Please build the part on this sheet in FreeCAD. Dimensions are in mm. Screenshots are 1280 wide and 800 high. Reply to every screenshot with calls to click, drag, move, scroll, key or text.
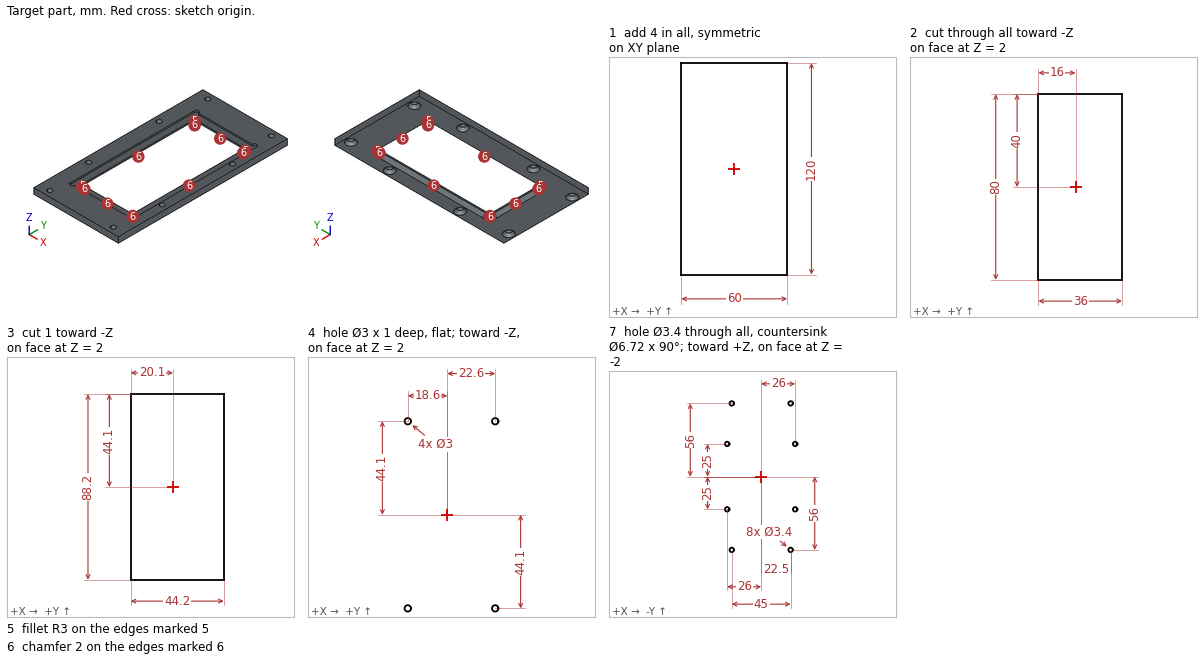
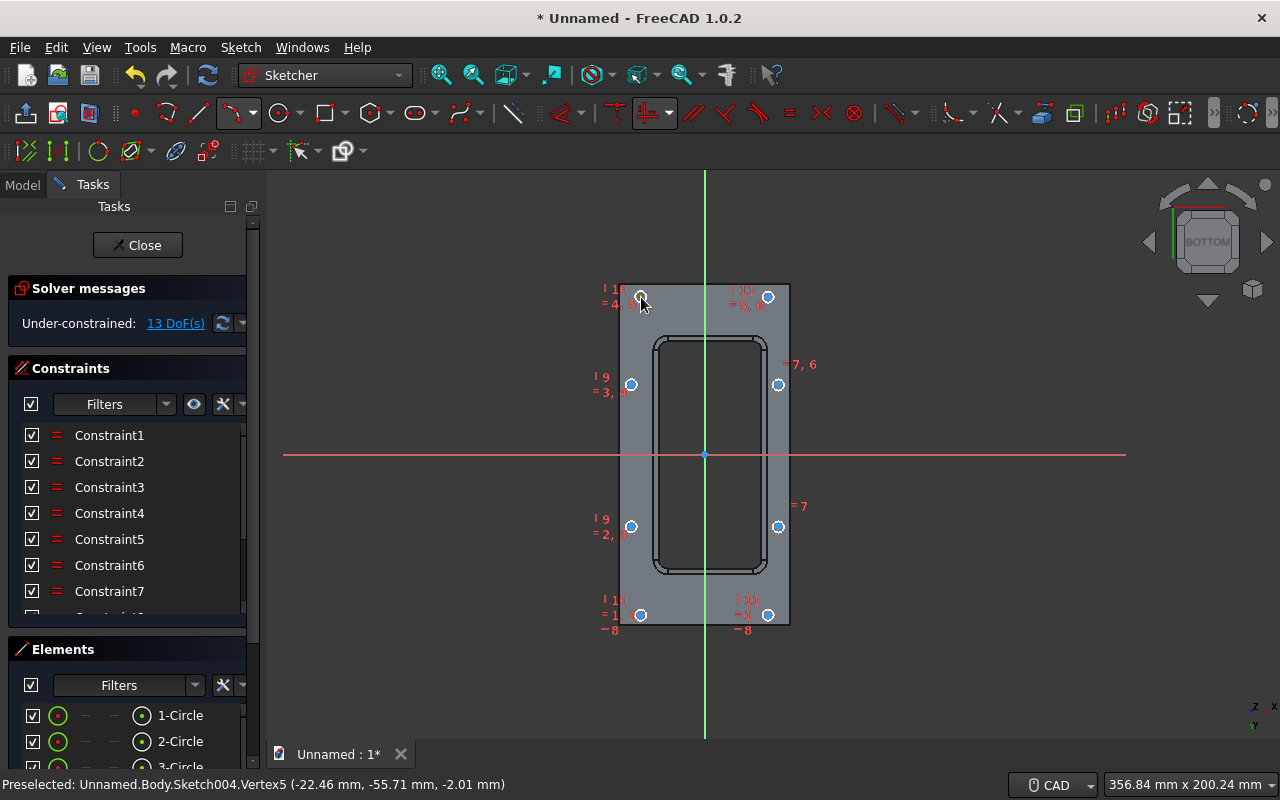
click(768, 297)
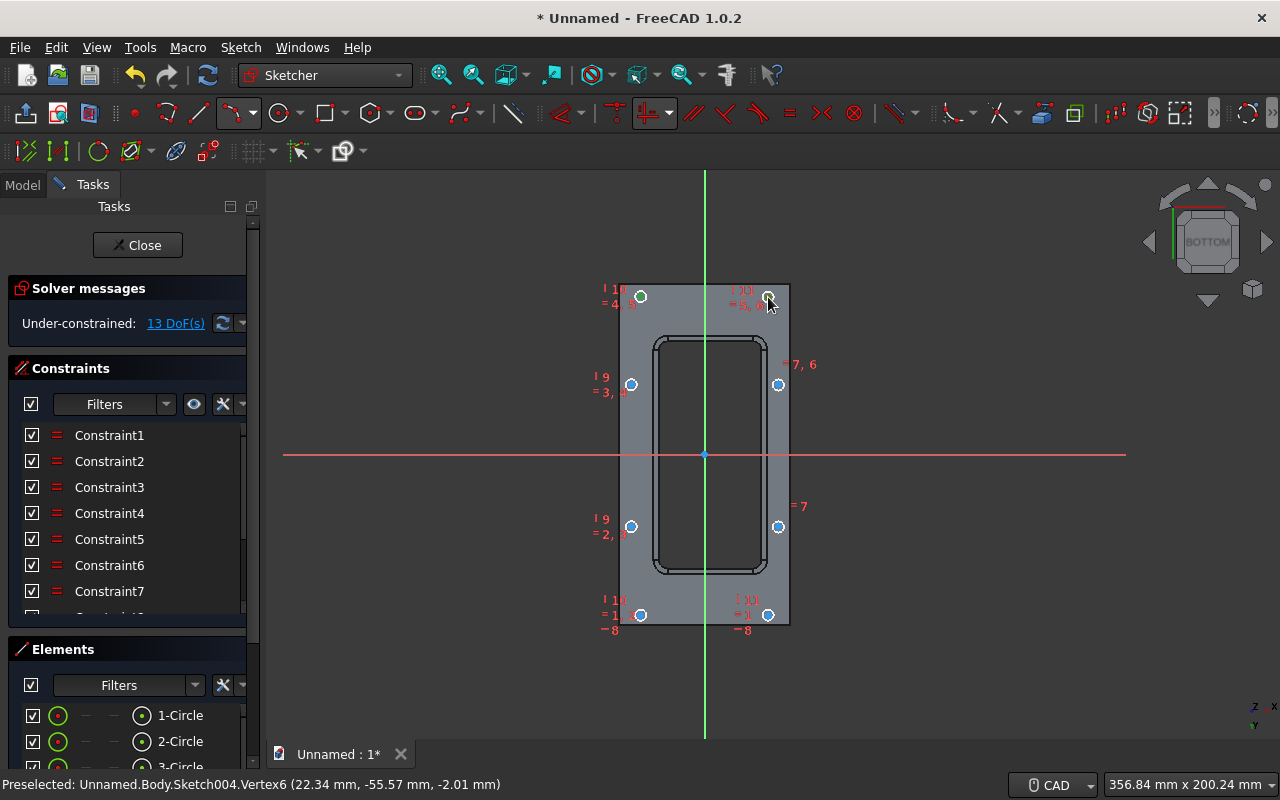
key(h)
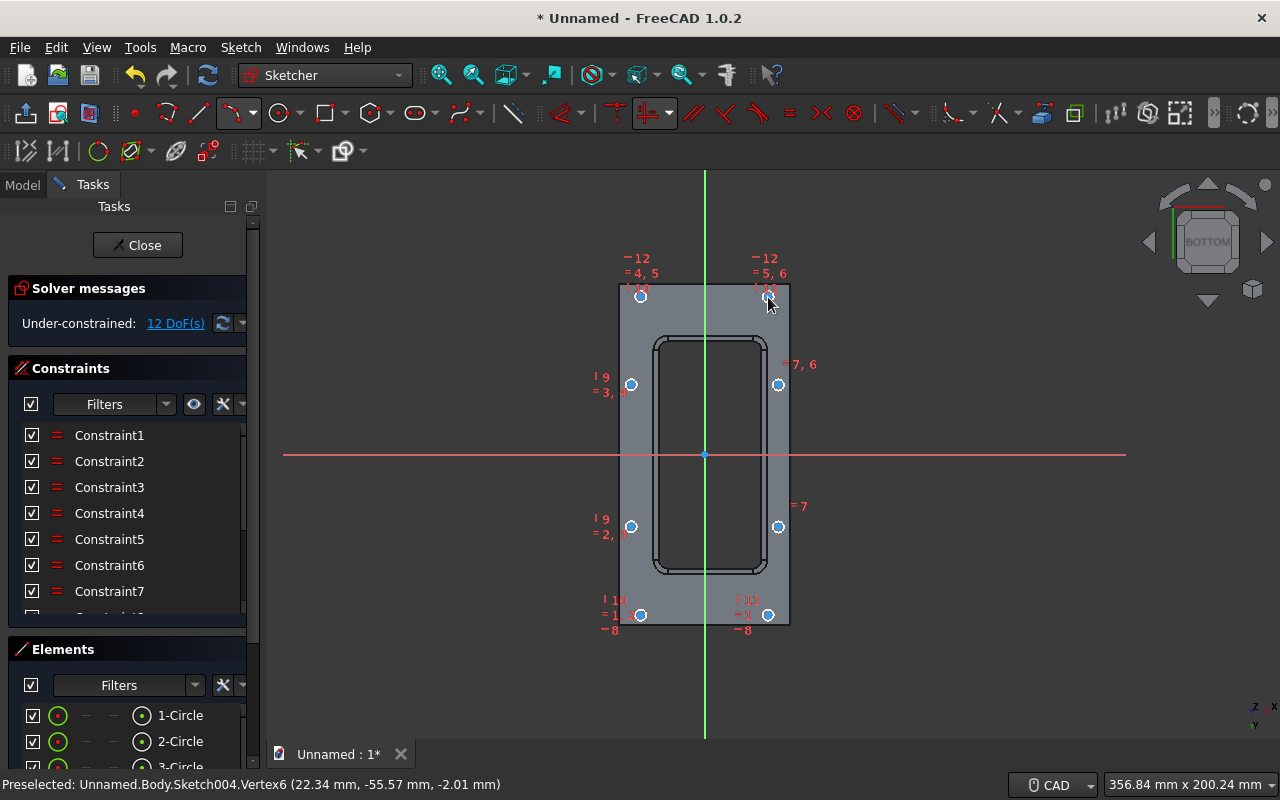
click(631, 385)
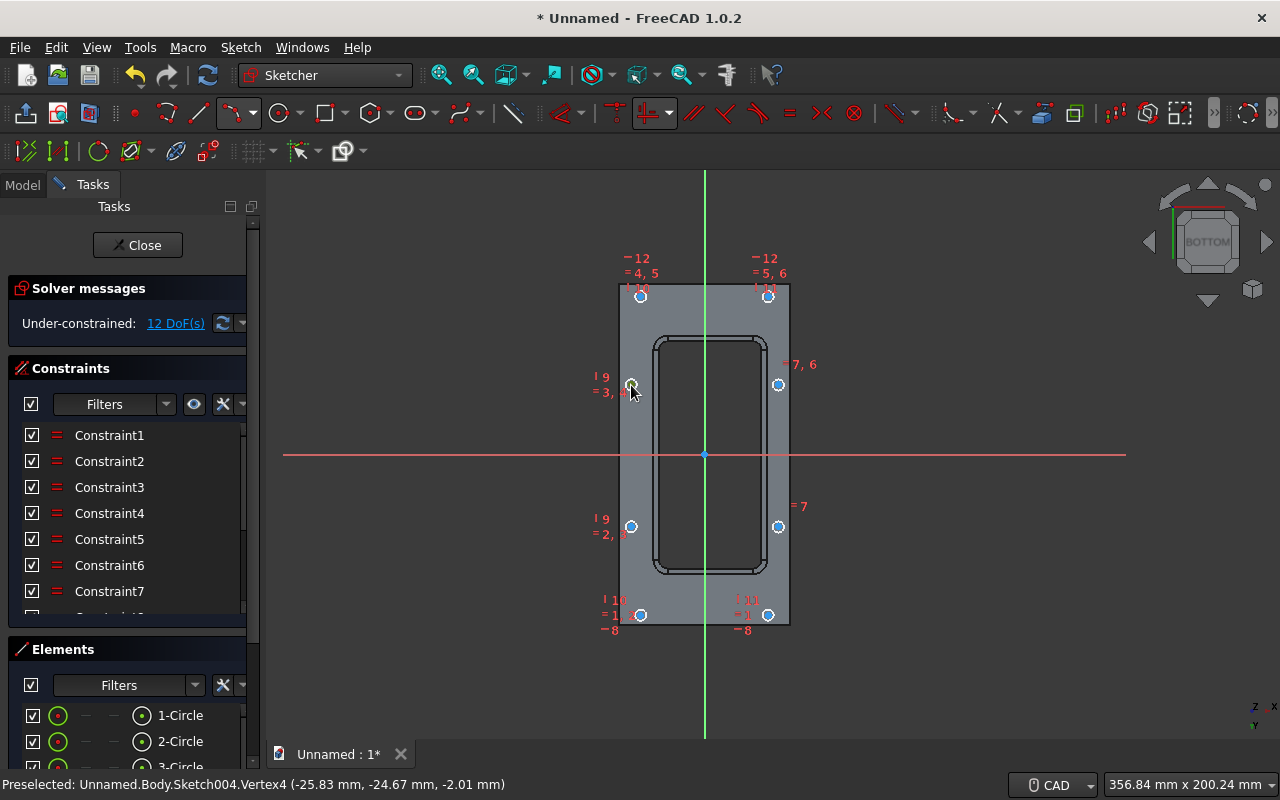
click(778, 385)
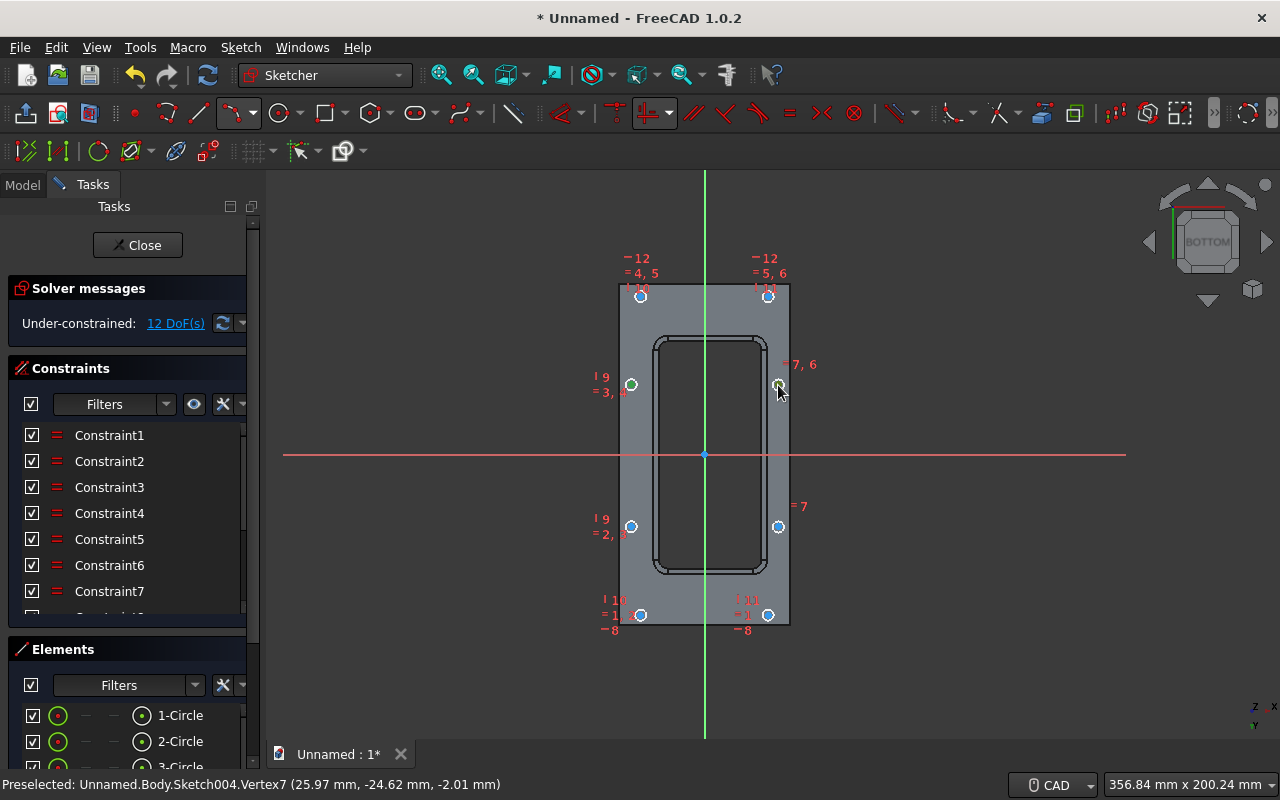
click(672, 114)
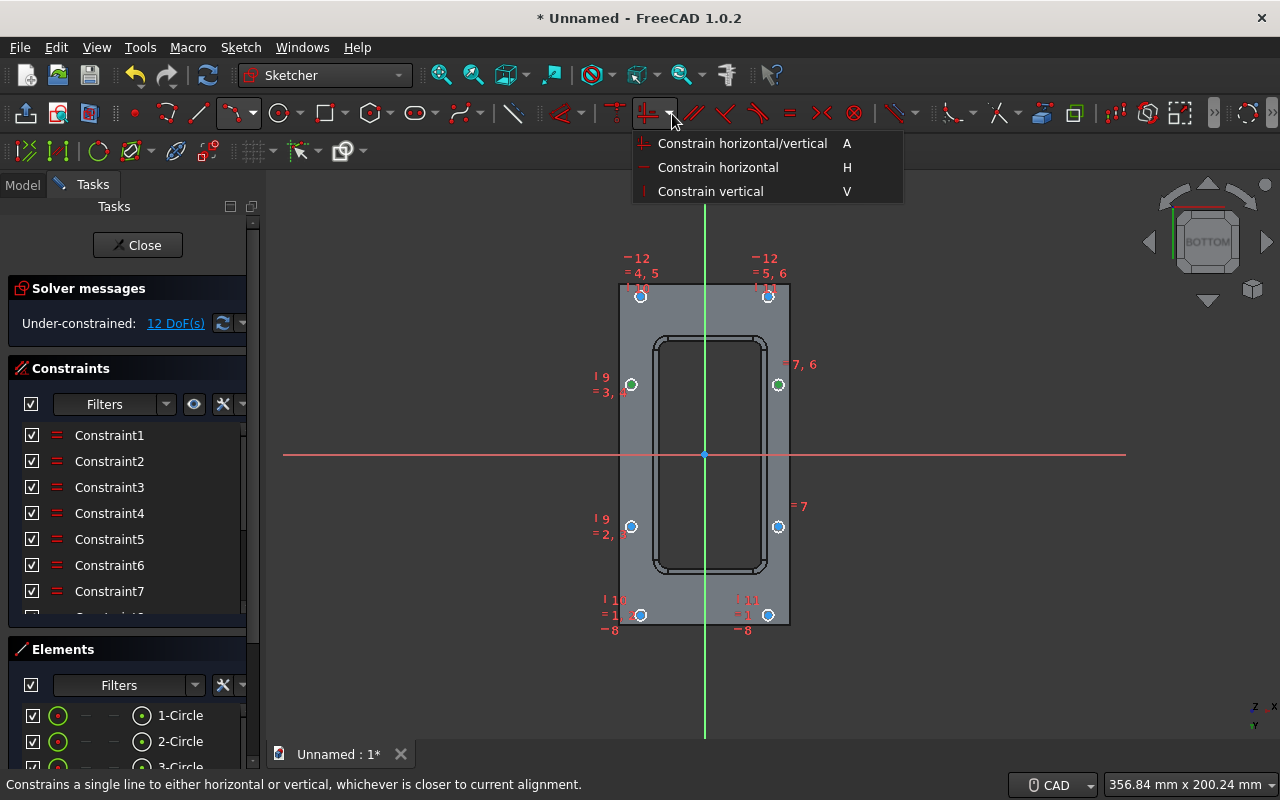
click(768, 167)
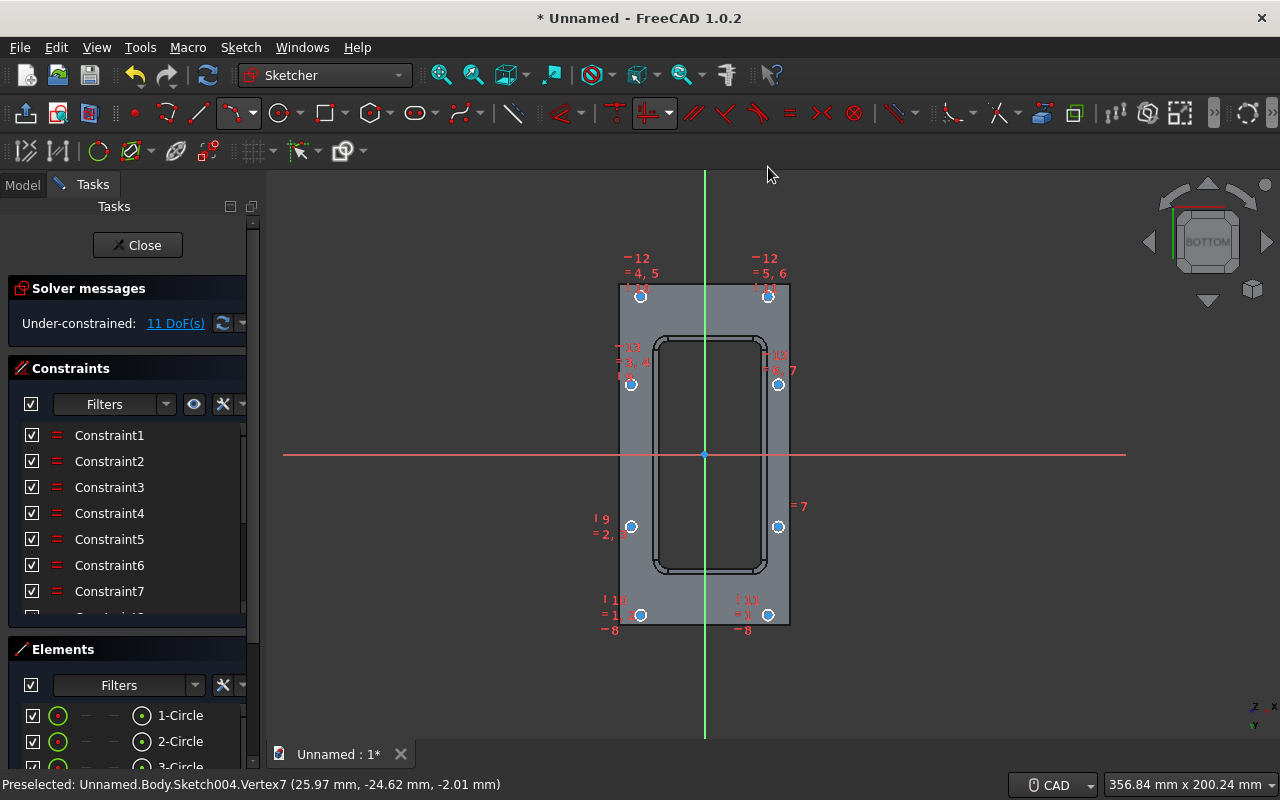
click(778, 385)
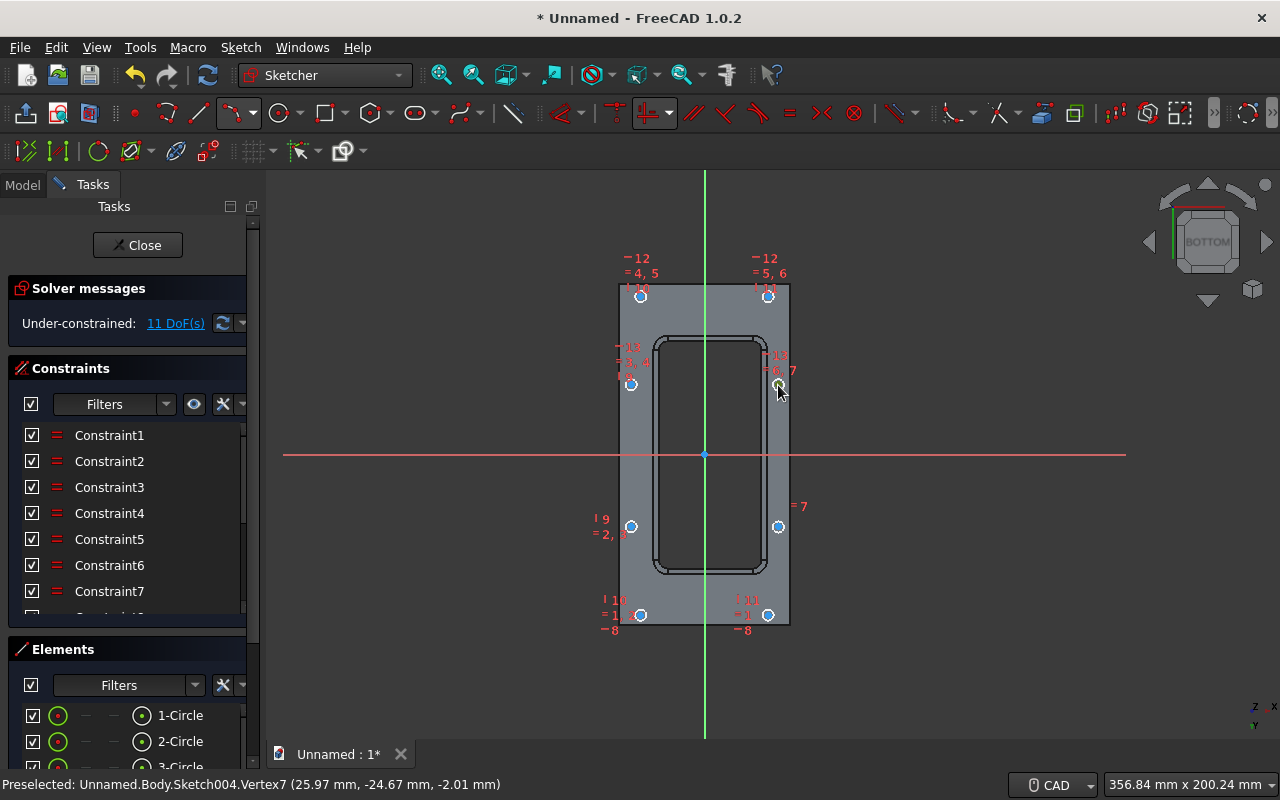
click(778, 527)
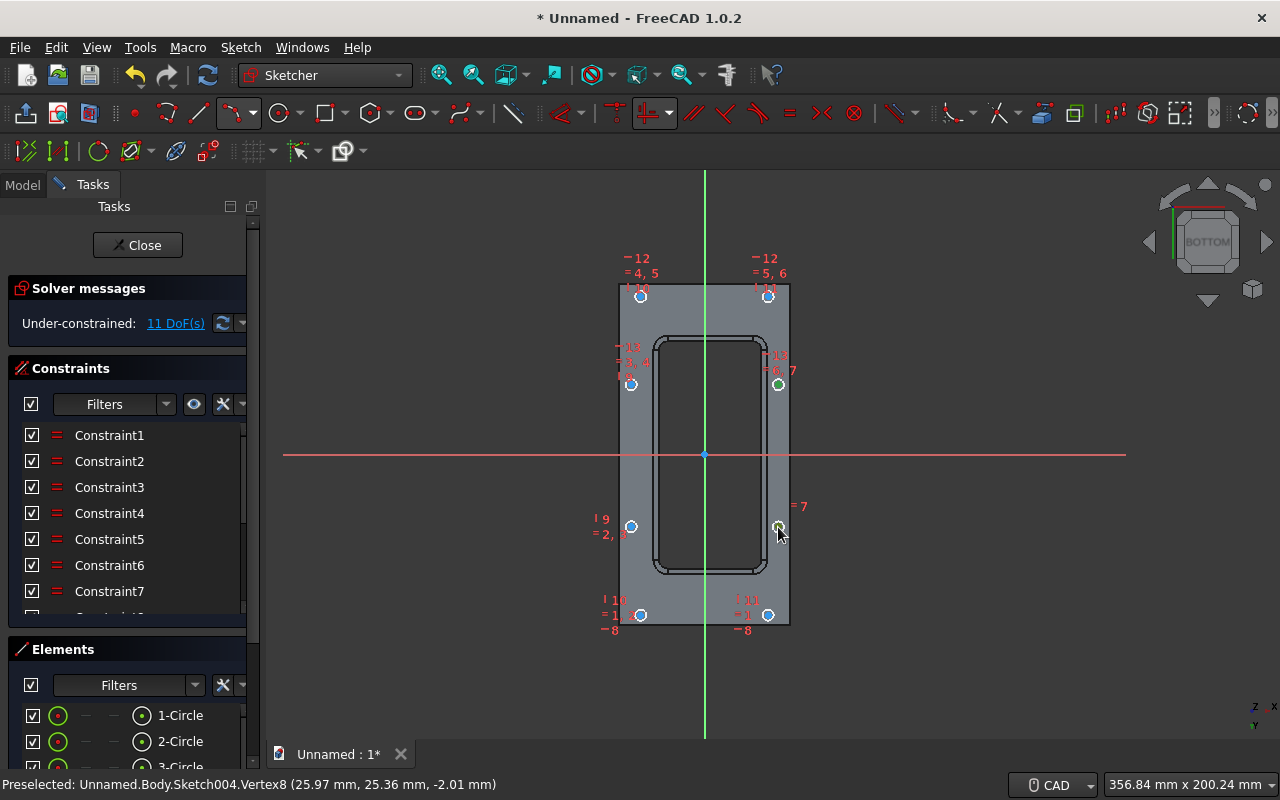
click(672, 114)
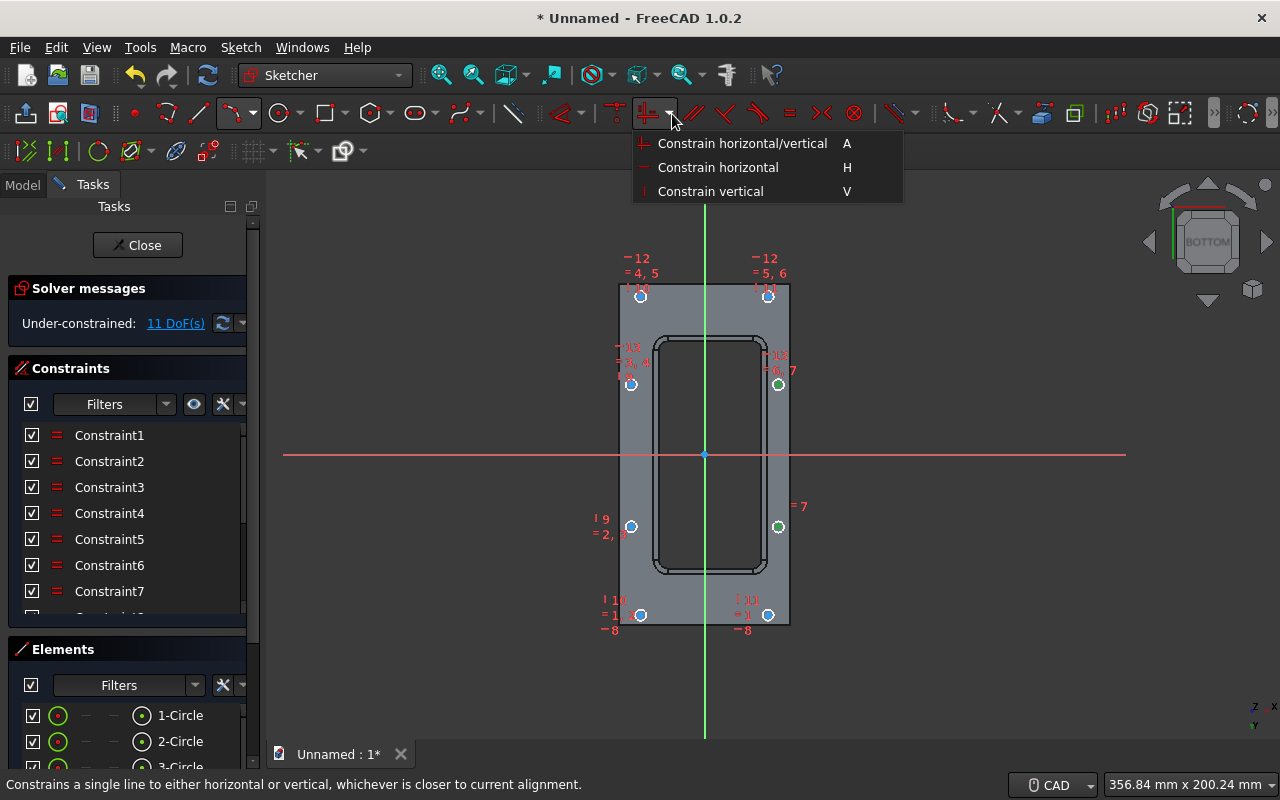
click(768, 191)